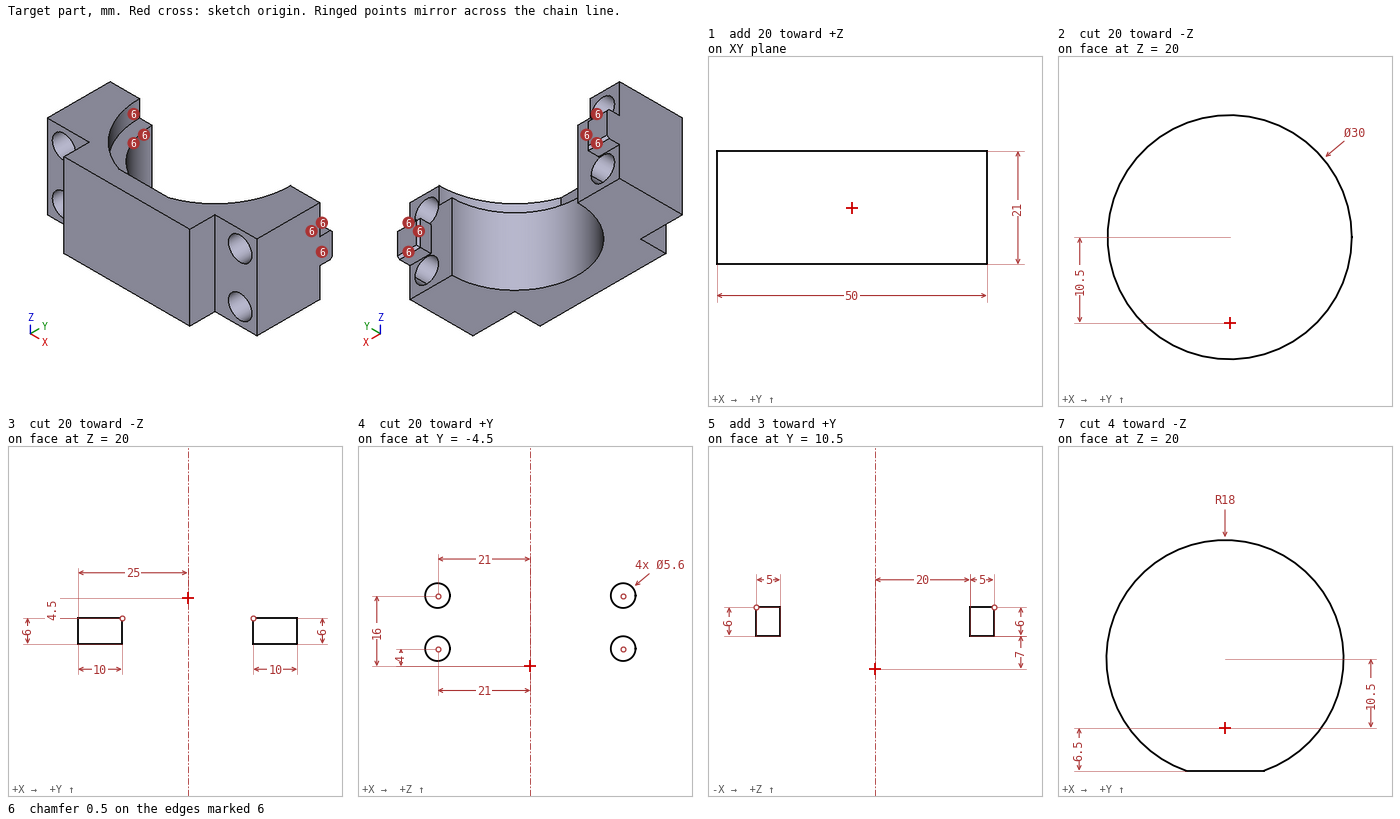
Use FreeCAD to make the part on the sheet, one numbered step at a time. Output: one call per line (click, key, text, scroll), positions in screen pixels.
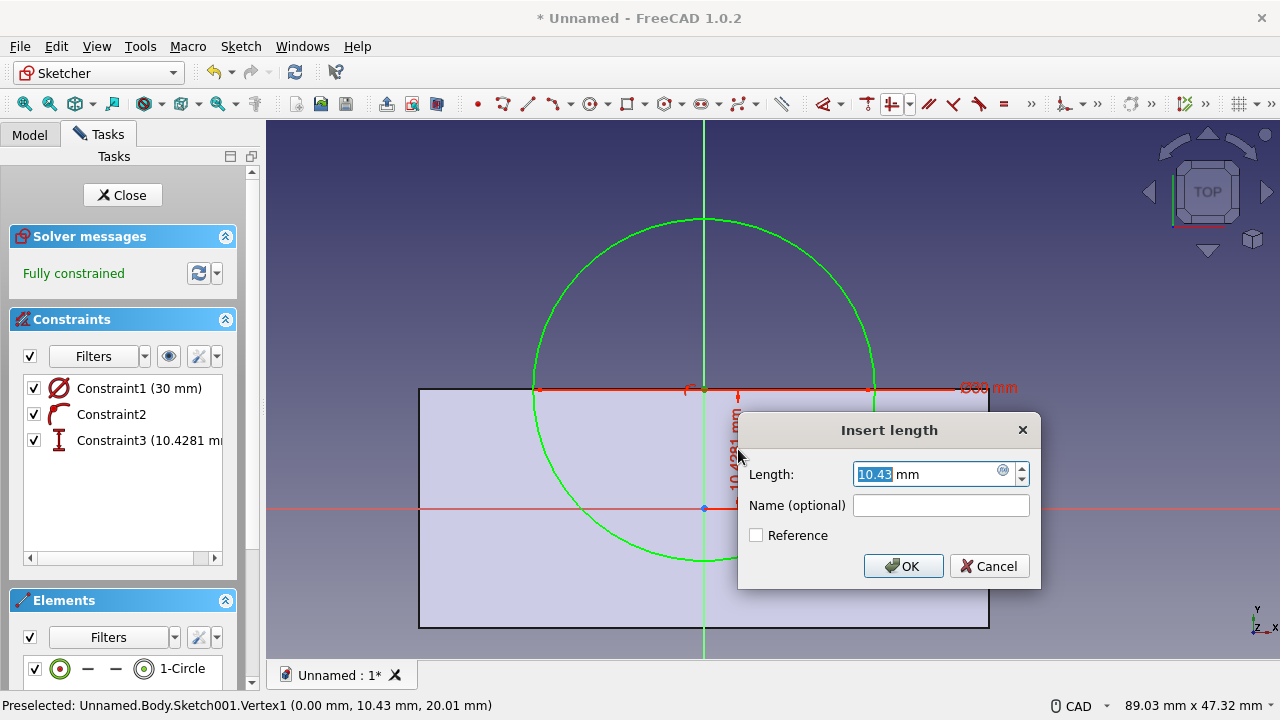
text(10.5)
key(Return)
key(Escape)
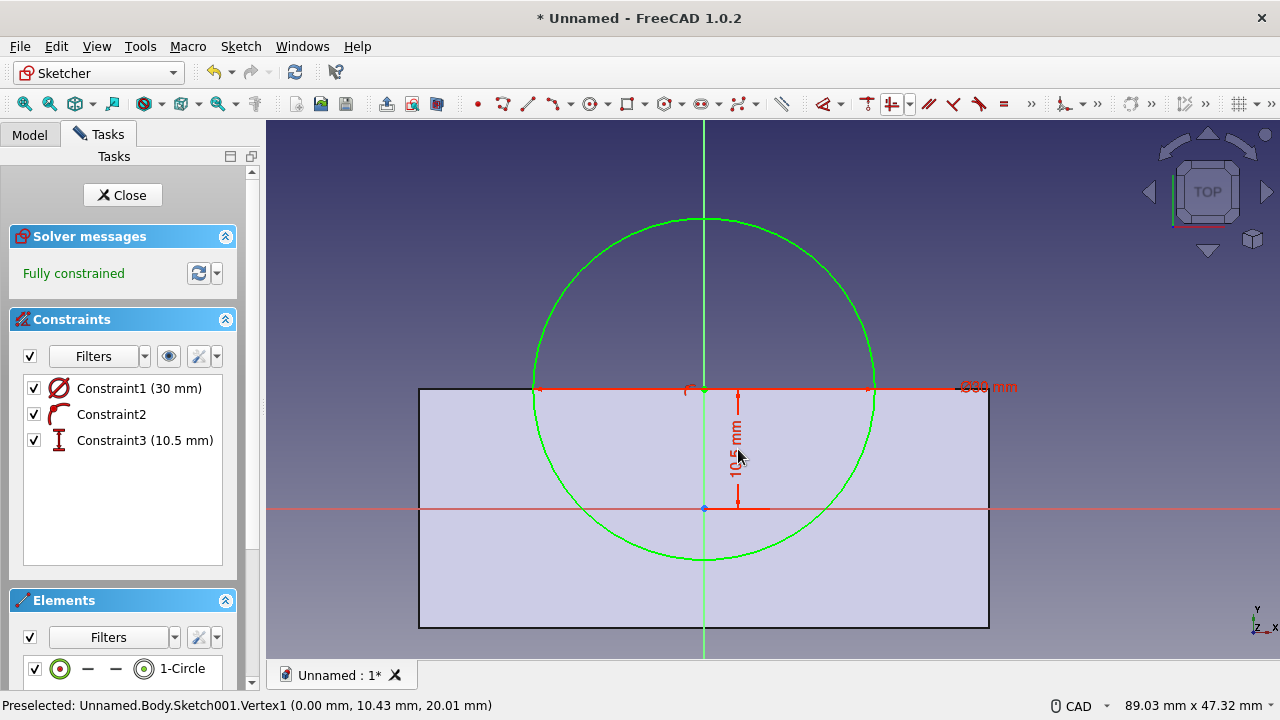
click(123, 195)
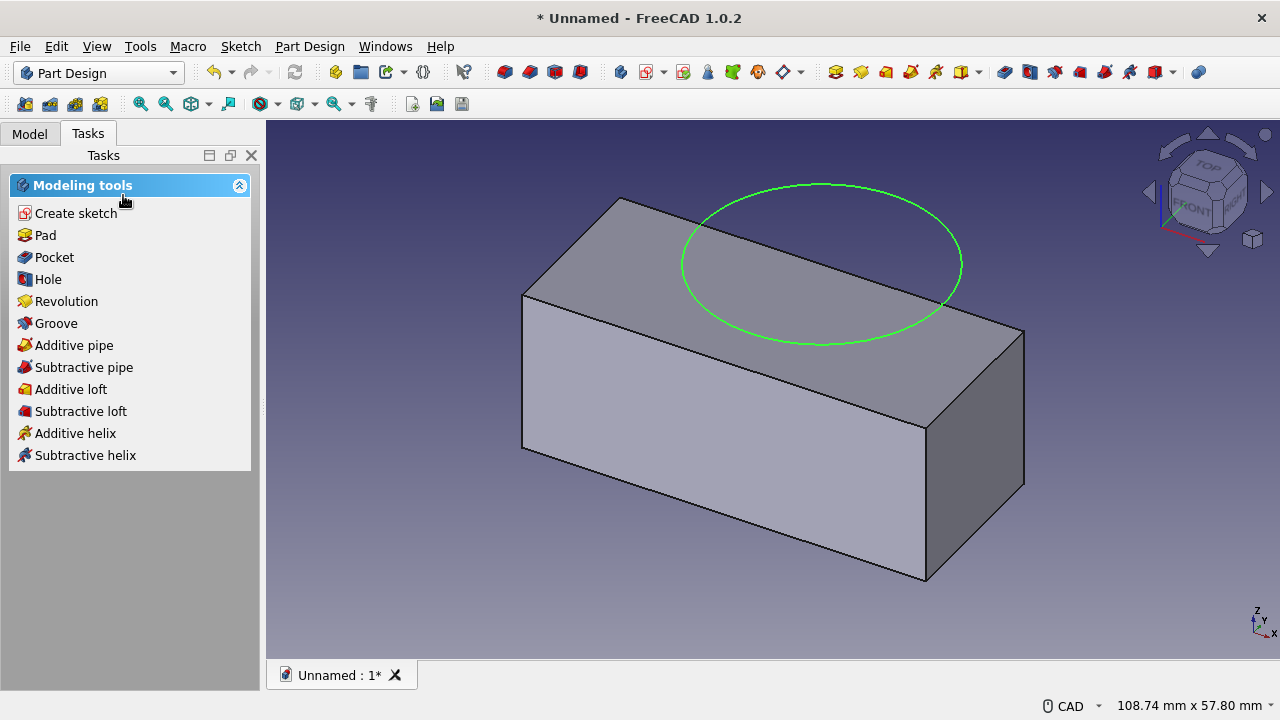
click(1005, 72)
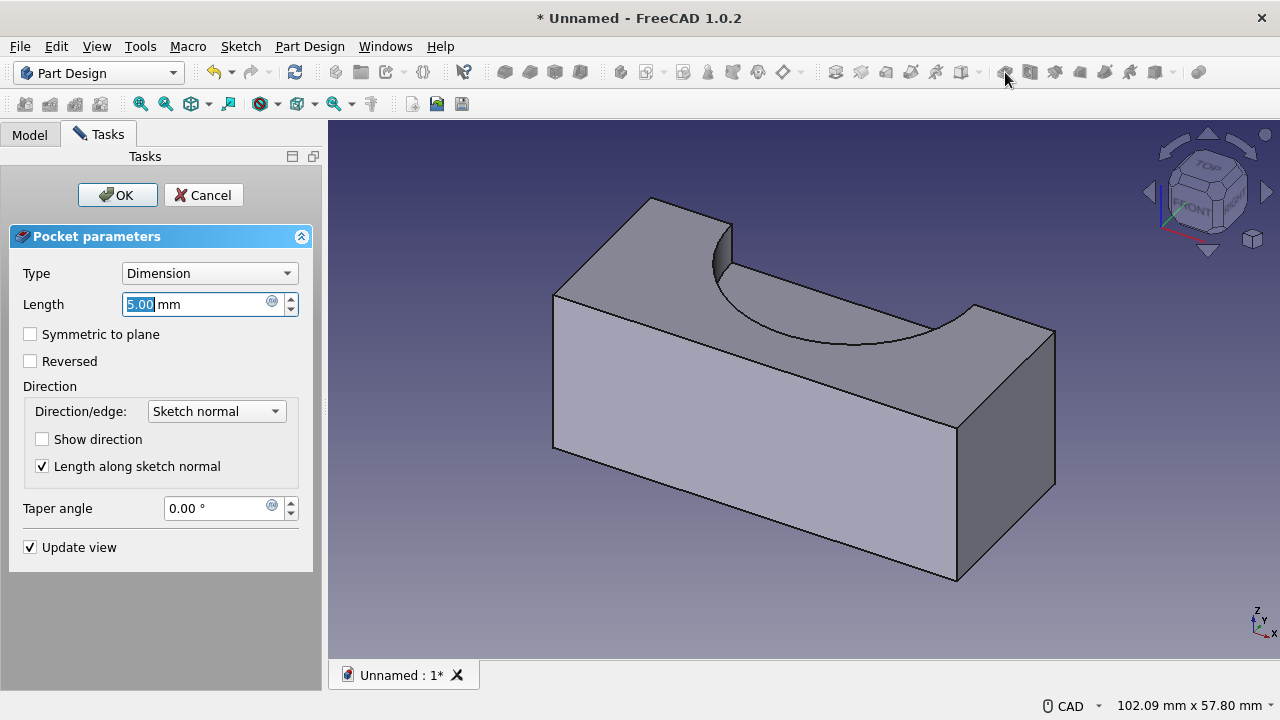
text(20)
key(Tab)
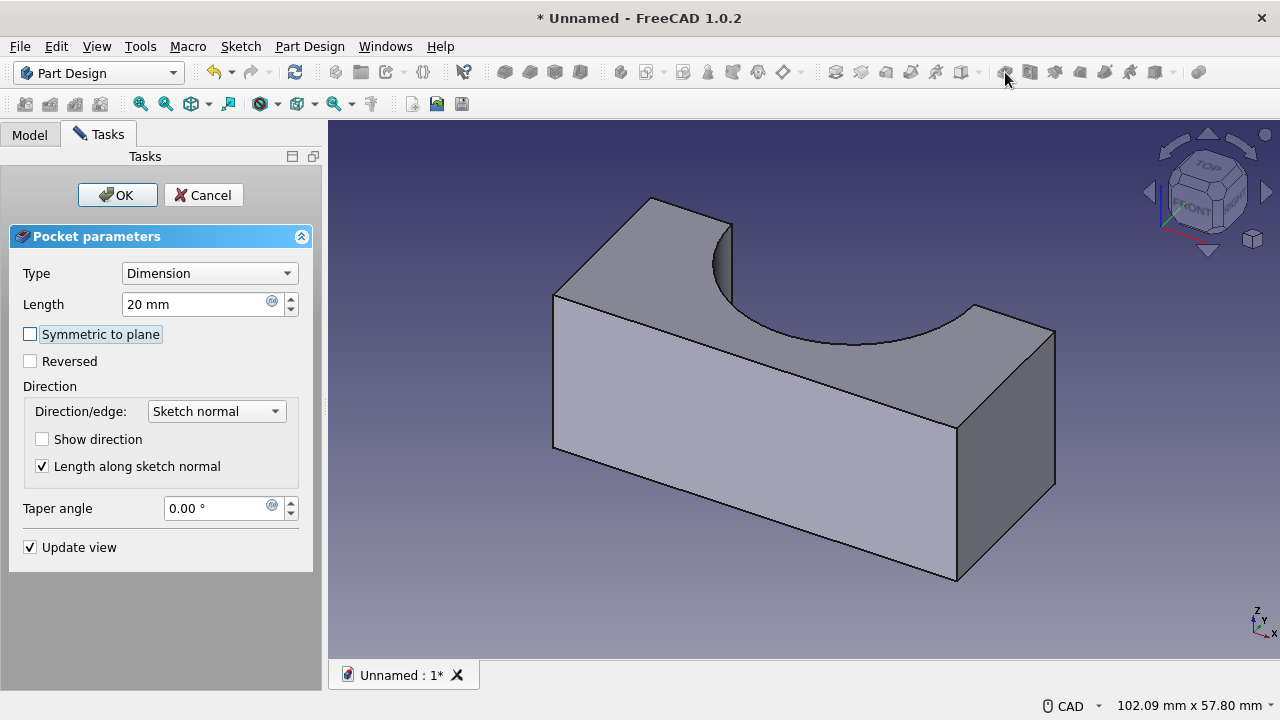
click(118, 195)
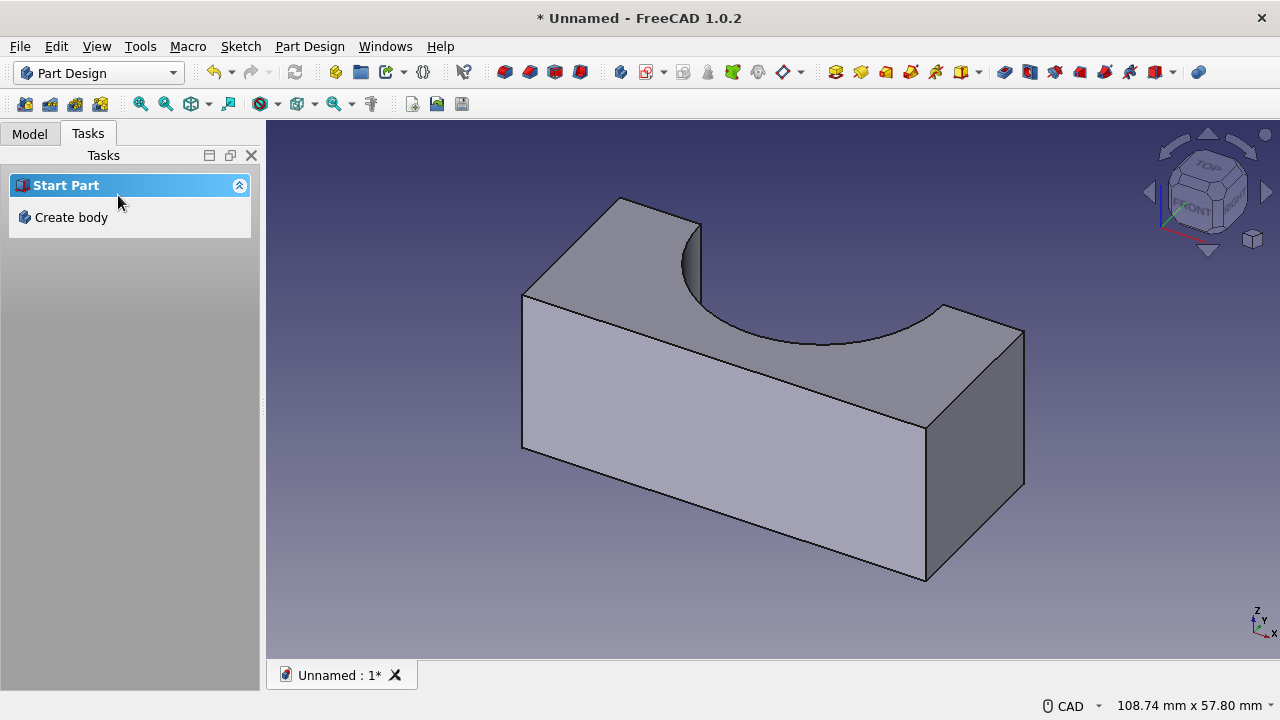
click(874, 364)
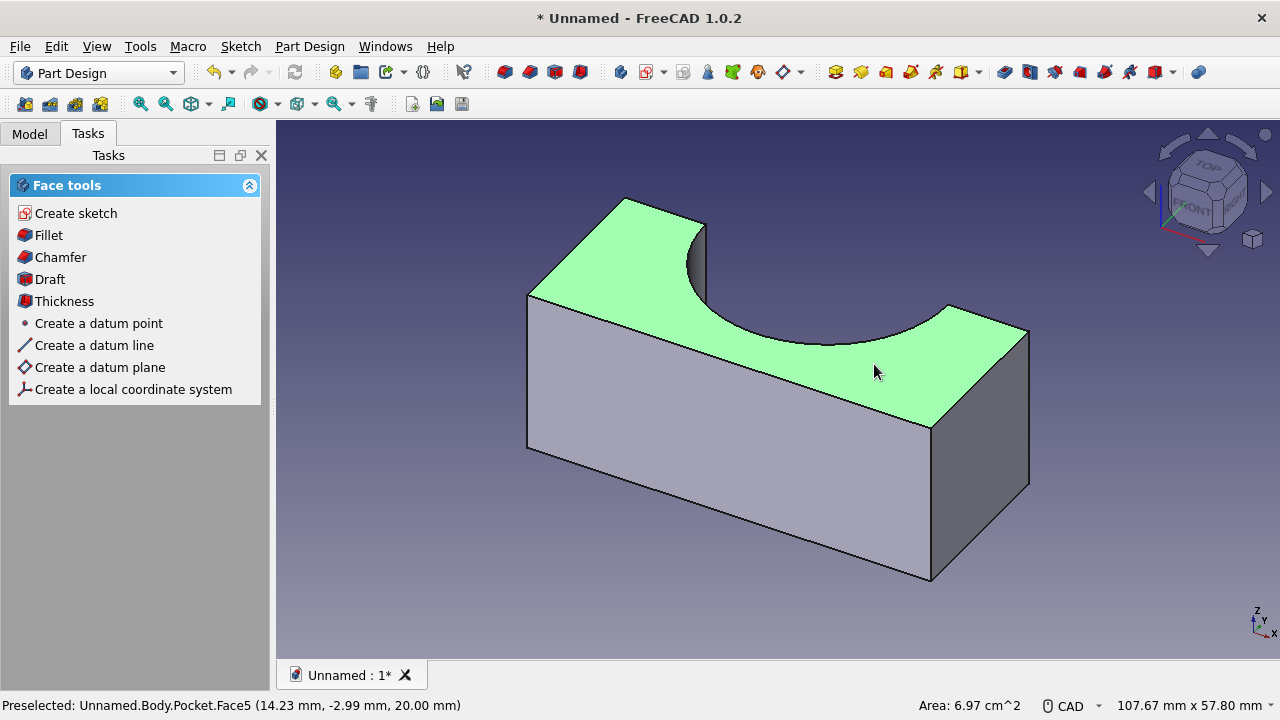
click(646, 72)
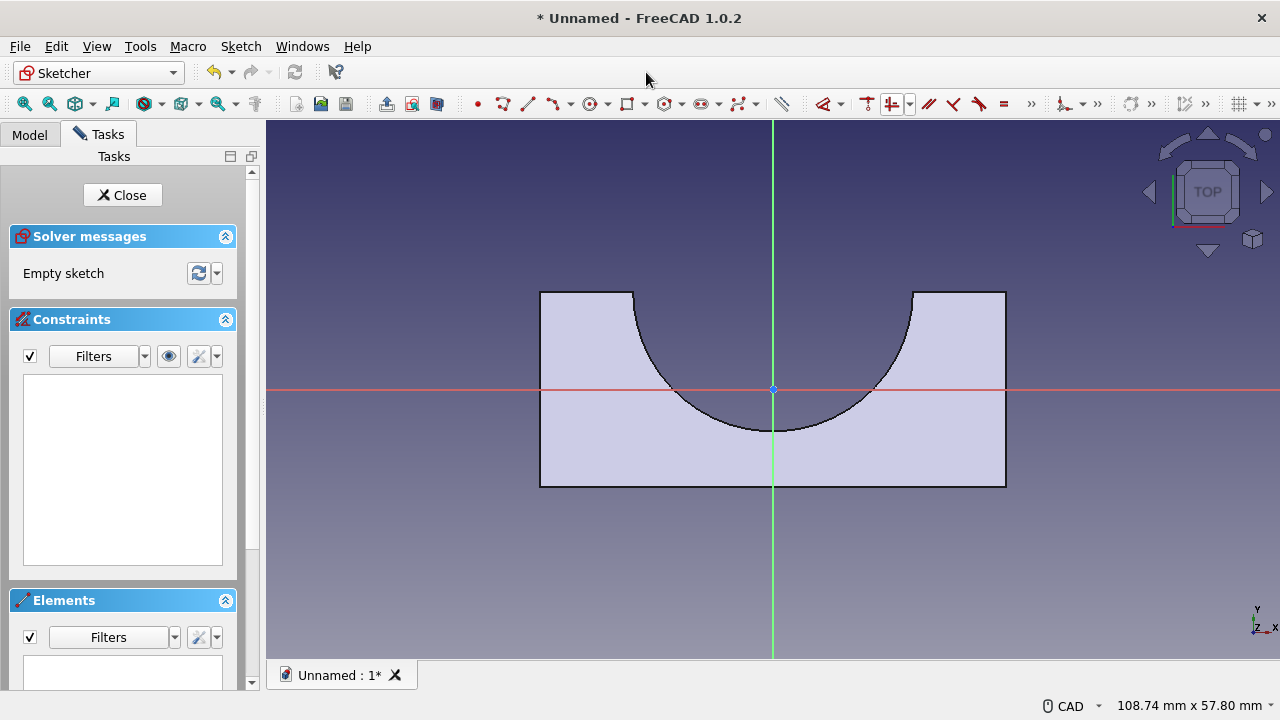
key(g)
key(r)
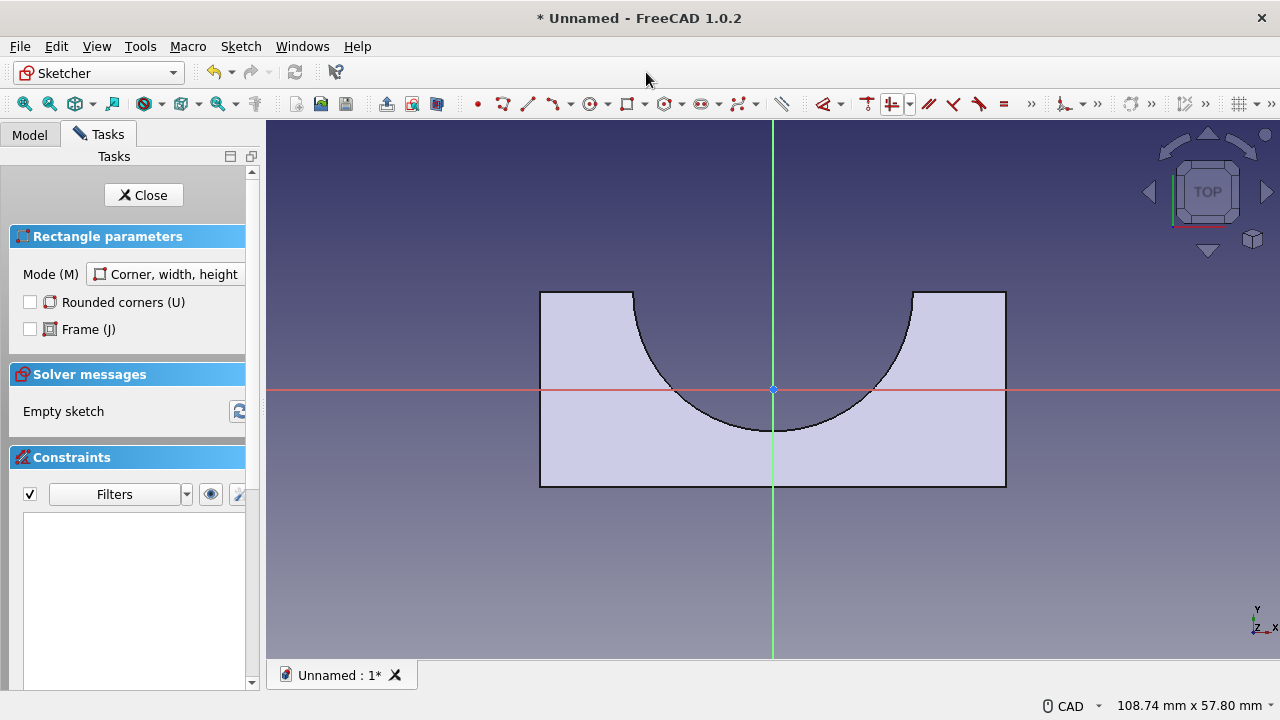
click(540, 431)
move(633, 487)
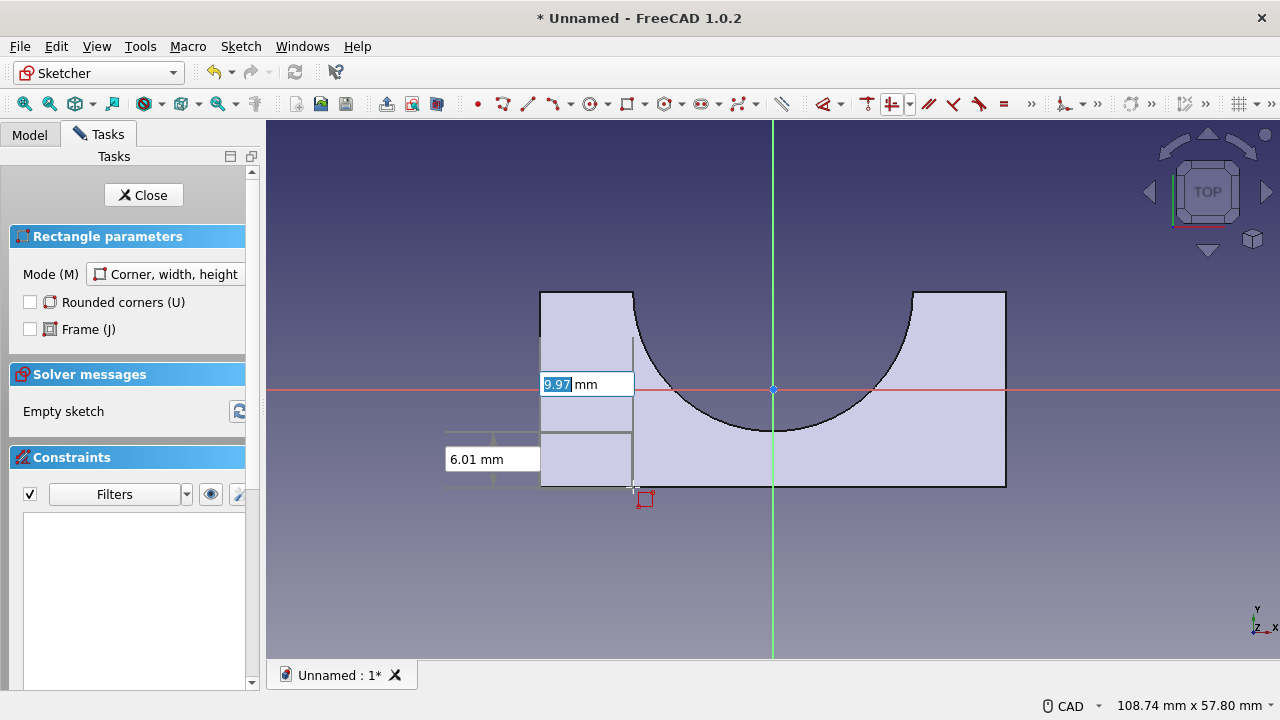
text(10)
key(Tab)
text(6)
key(Return)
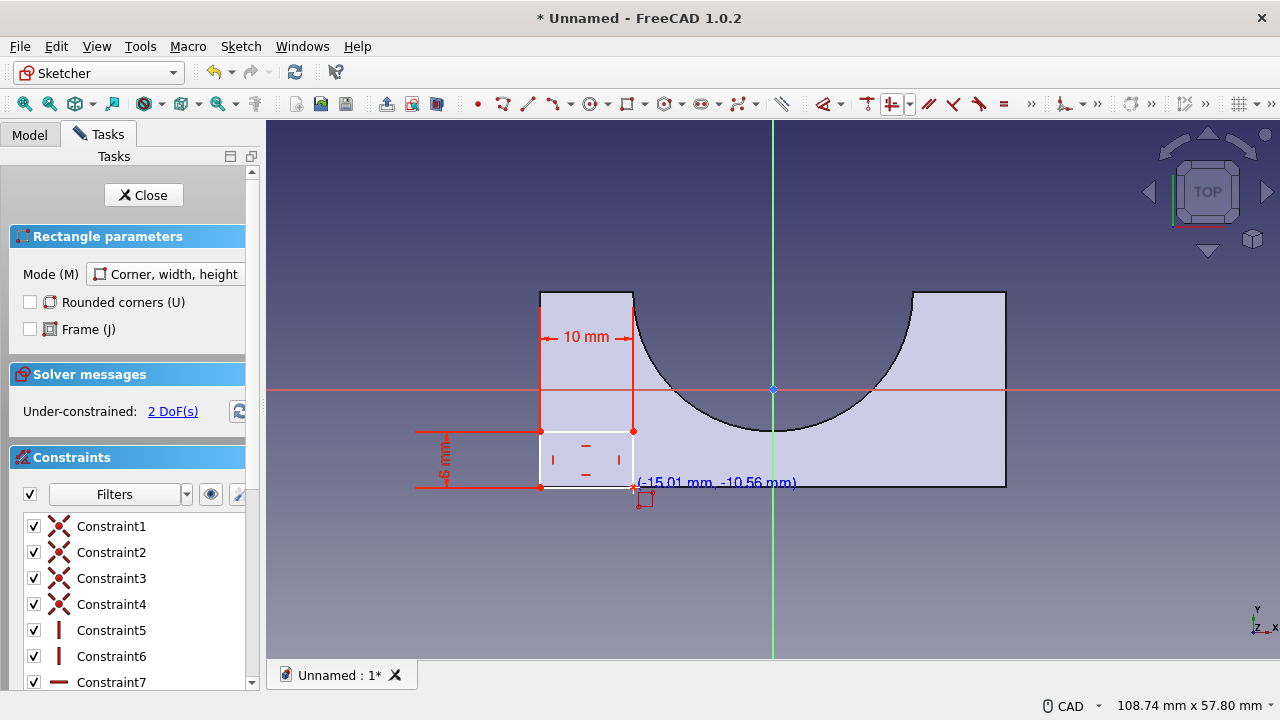
click(913, 431)
move(1006, 487)